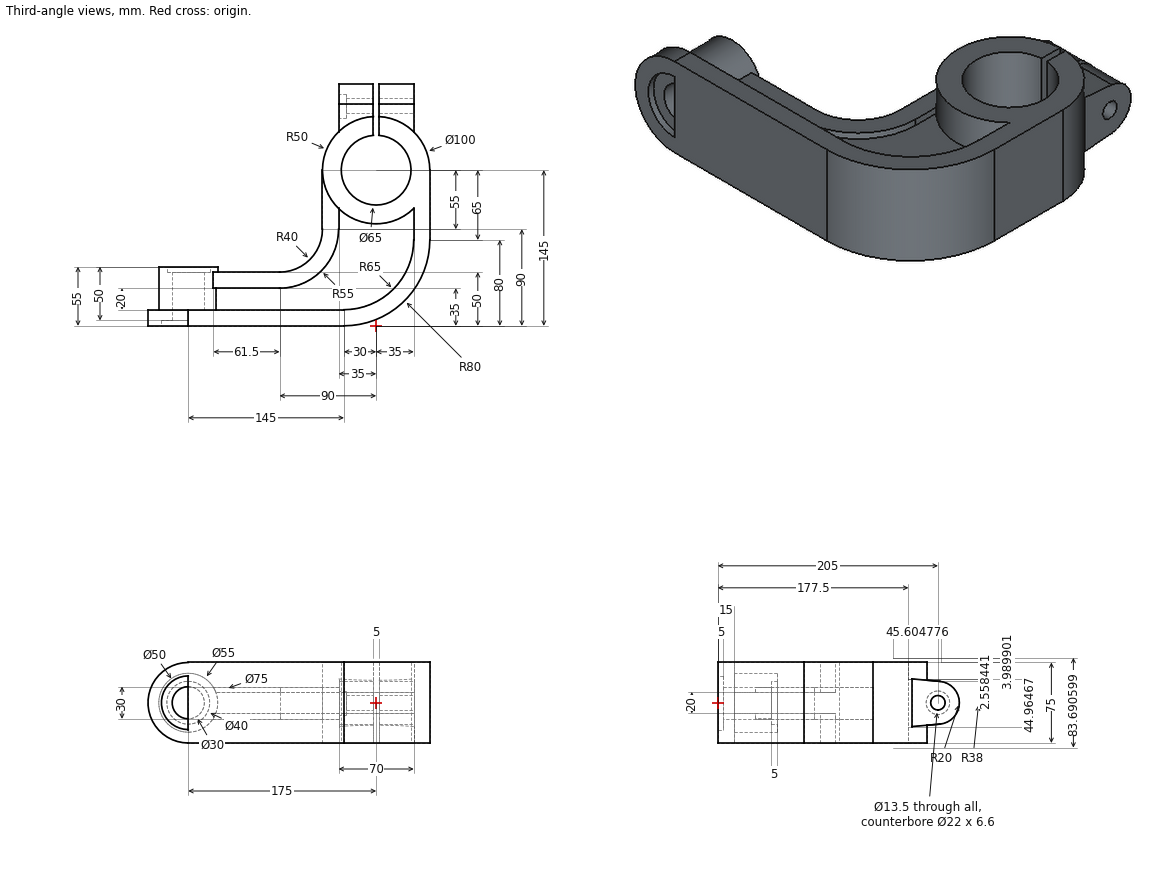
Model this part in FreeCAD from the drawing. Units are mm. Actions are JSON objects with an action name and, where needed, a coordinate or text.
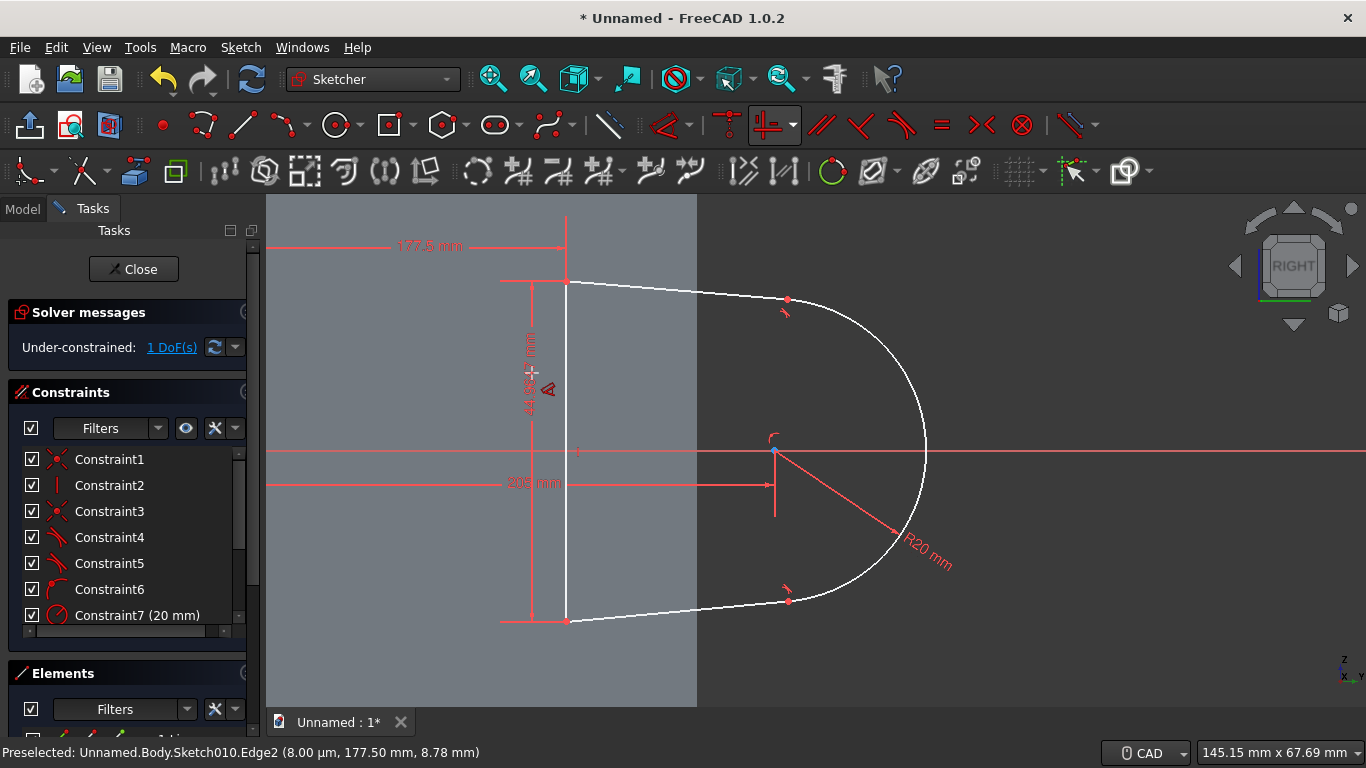
{"action": "scroll", "coordinate": [721, 294], "scroll_direction": "up", "scroll_amount": 4}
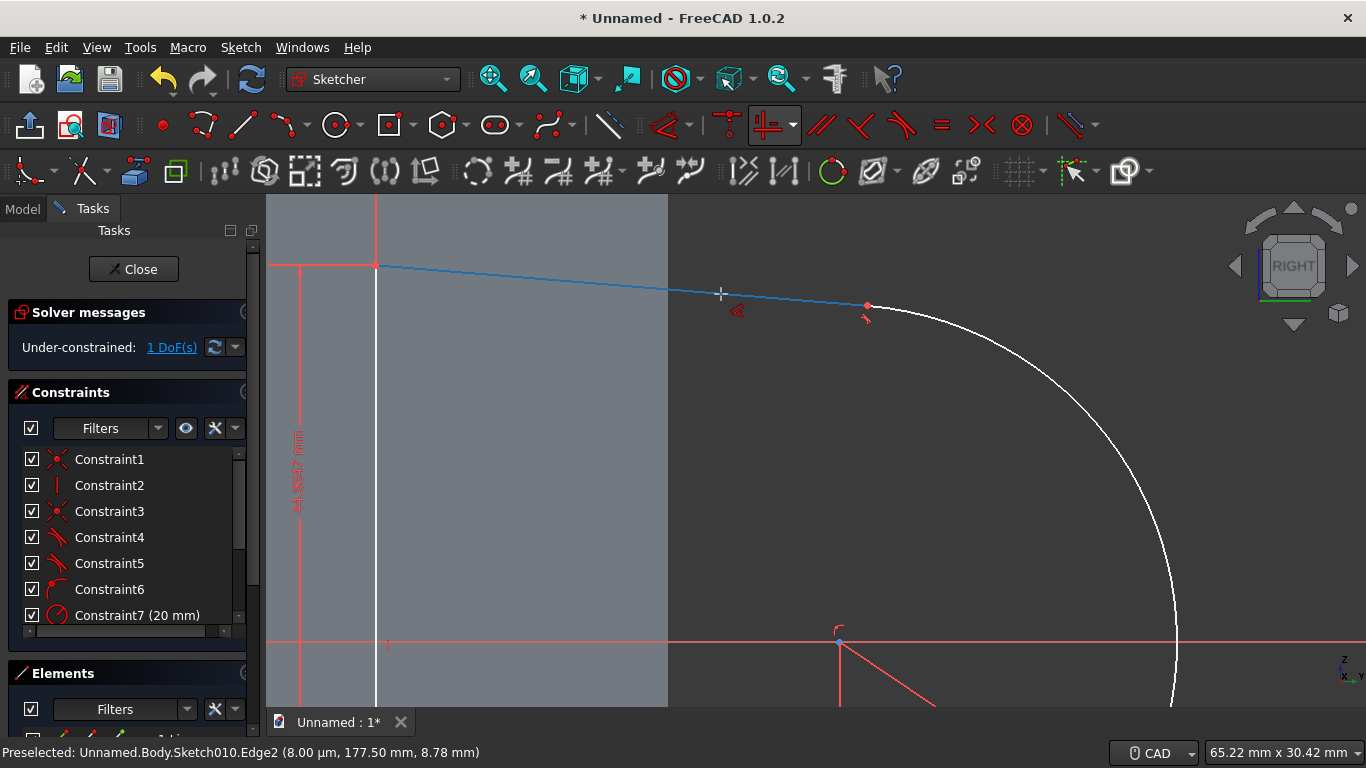
{"action": "left_click", "coordinate": [720, 294]}
{"action": "left_click", "coordinate": [342, 286]}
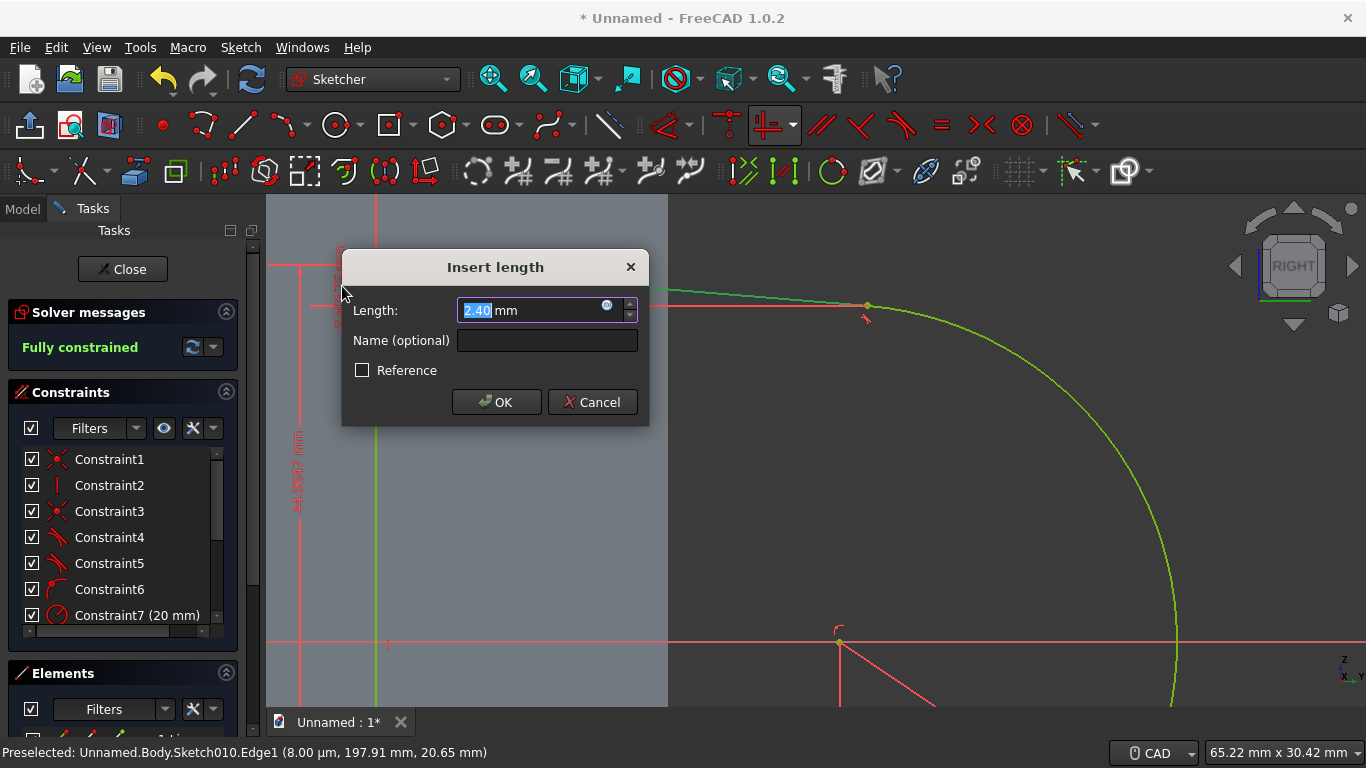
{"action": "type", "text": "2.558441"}
{"action": "key", "text": "Return"}
{"action": "key", "text": "Escape"}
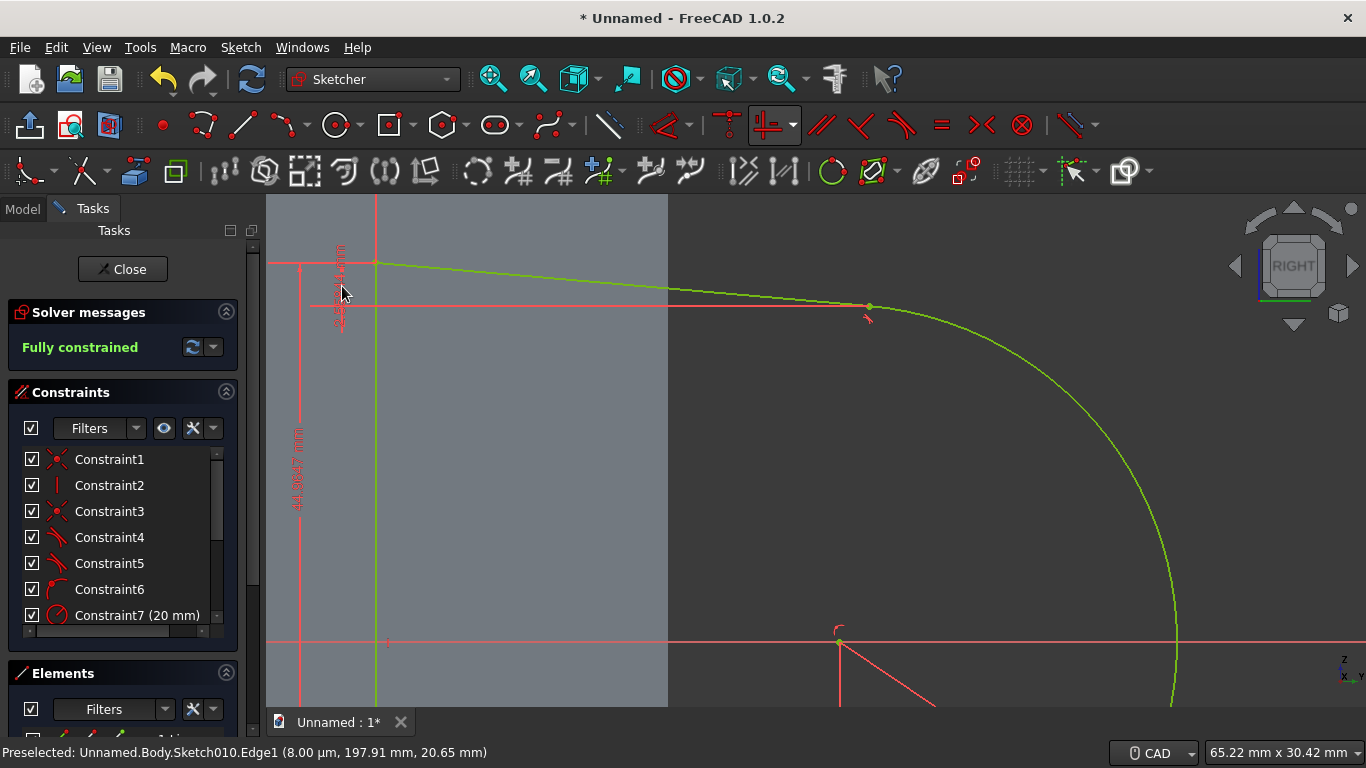
{"action": "left_click", "coordinate": [123, 269]}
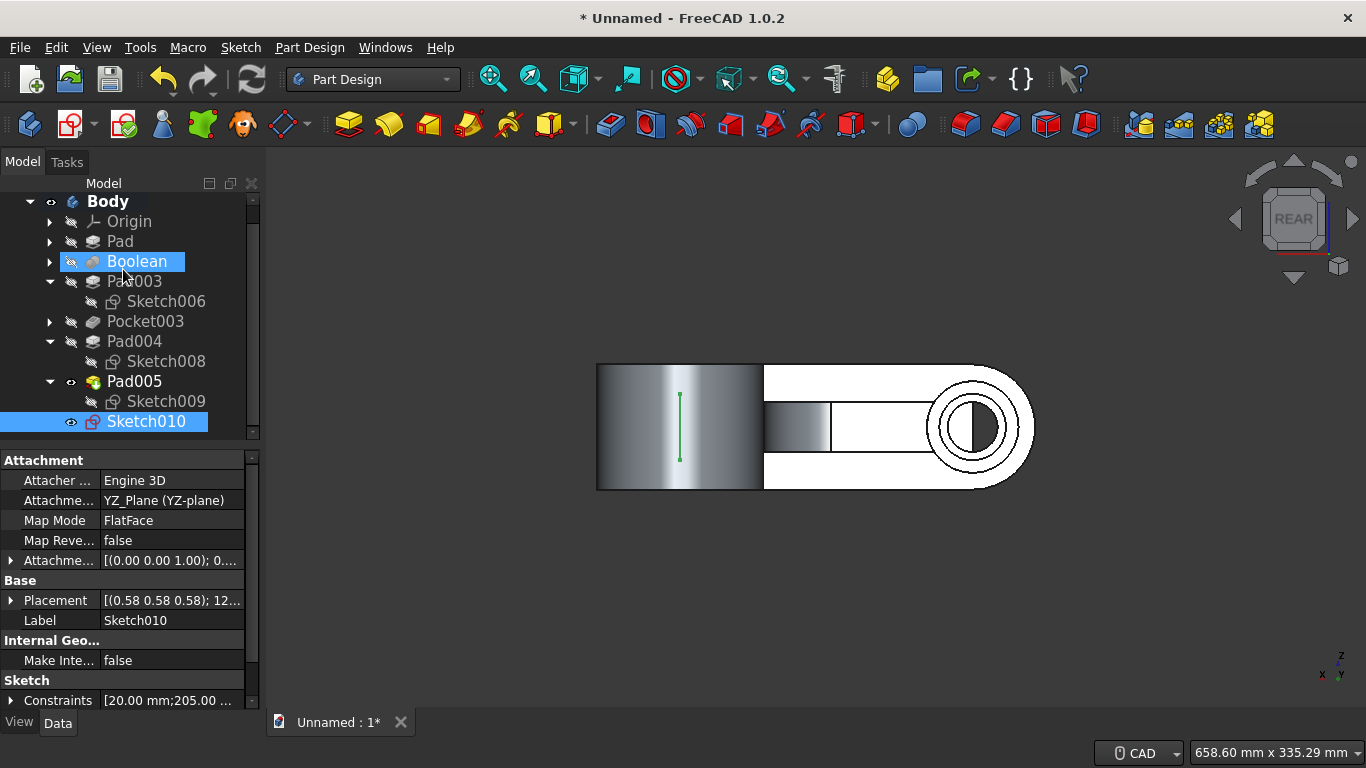
{"action": "left_click", "coordinate": [350, 124]}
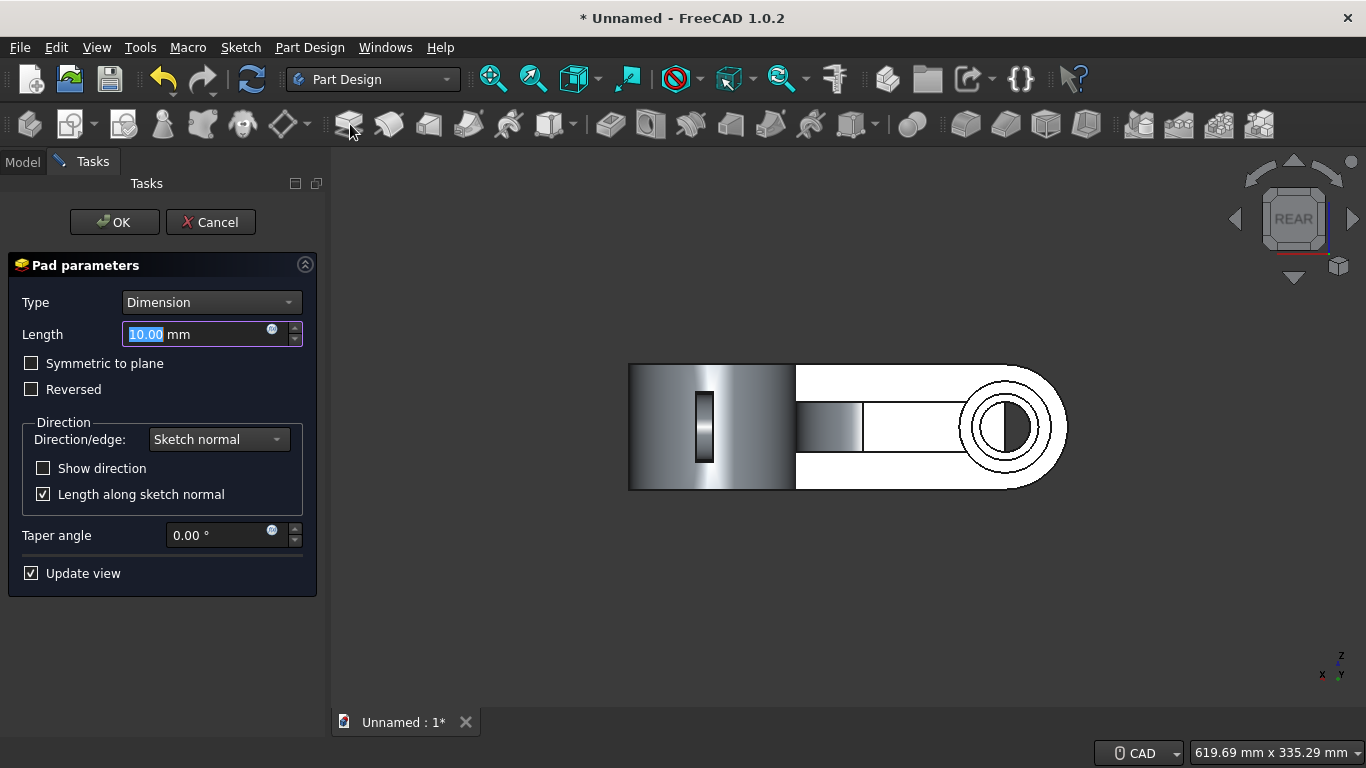
{"action": "type", "text": "70"}
{"action": "key", "text": "Tab"}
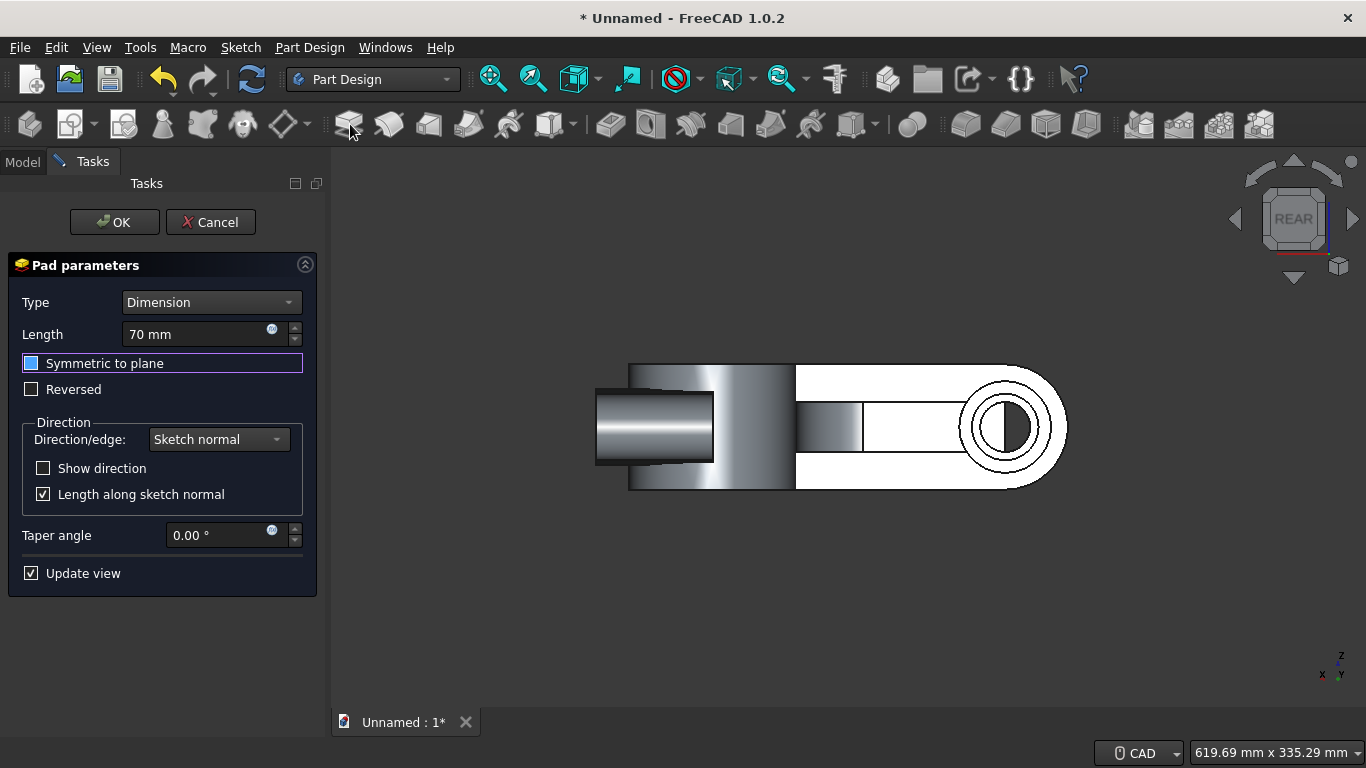
{"action": "left_click", "coordinate": [30, 363]}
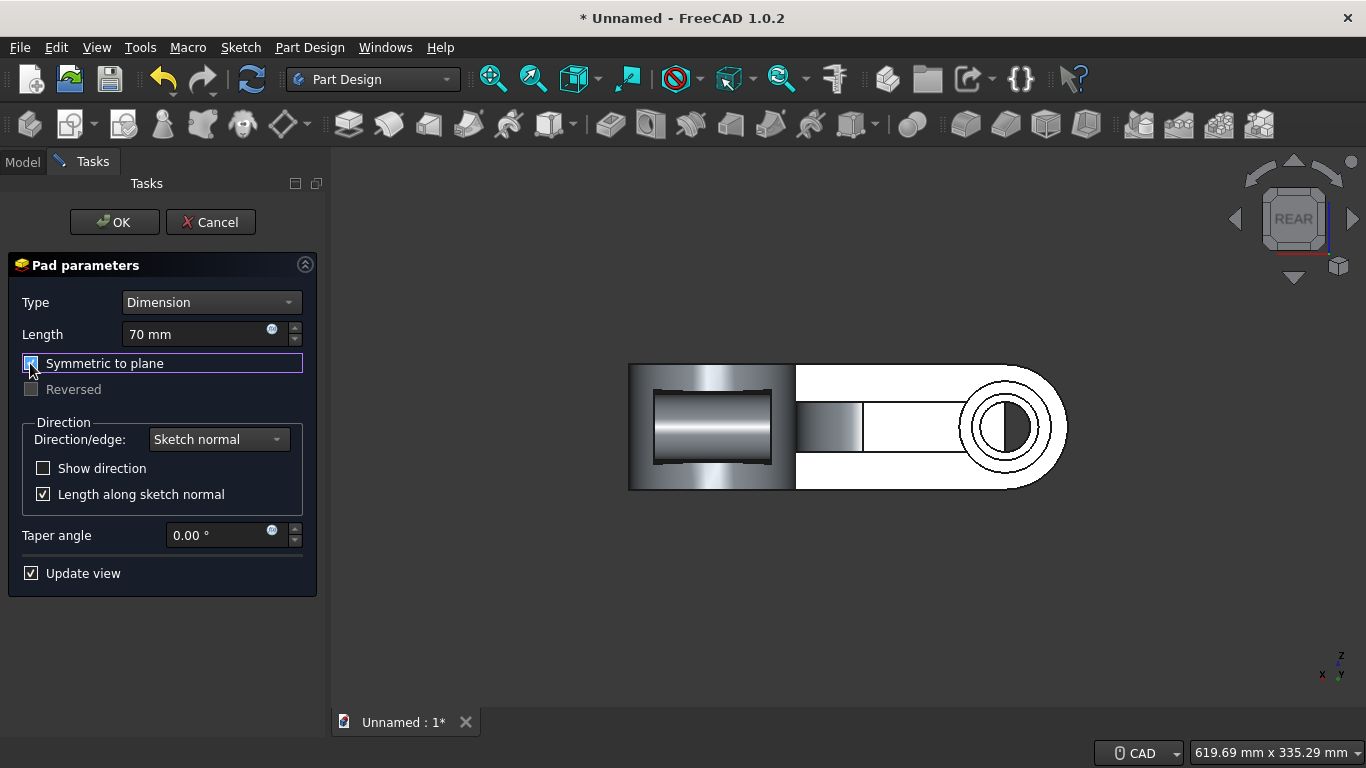
{"action": "left_click", "coordinate": [115, 222]}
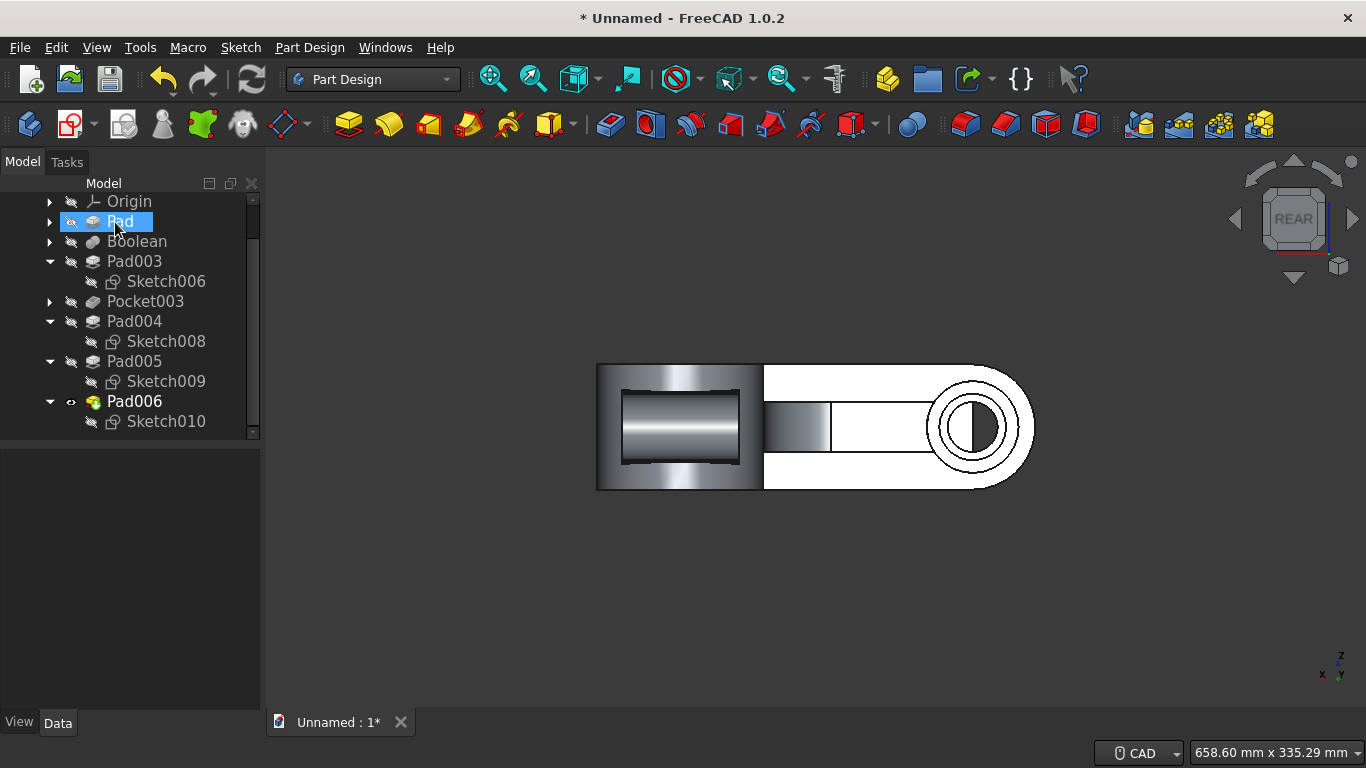
{"action": "key", "text": "v f"}